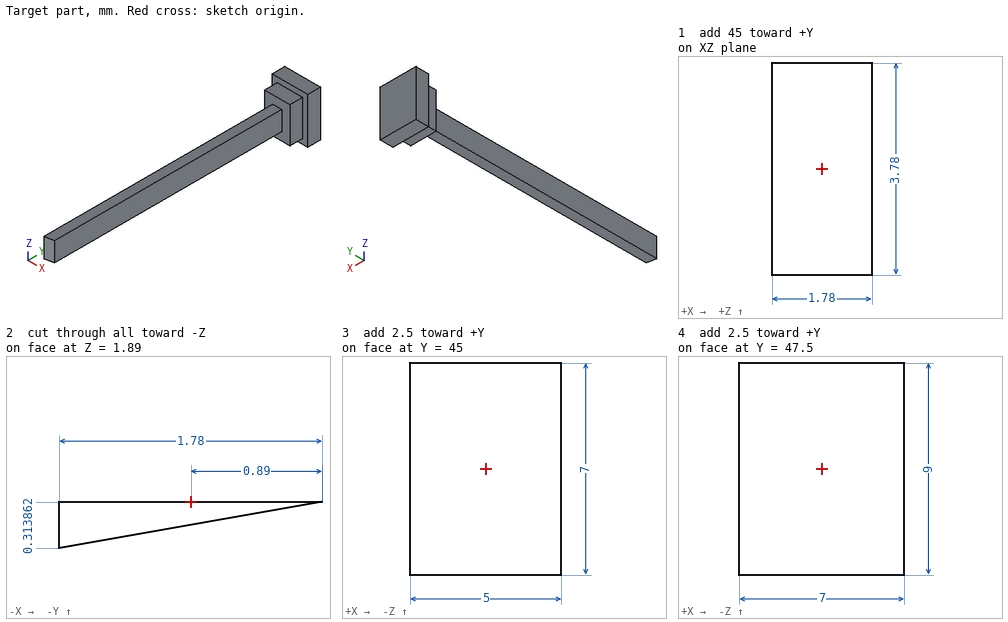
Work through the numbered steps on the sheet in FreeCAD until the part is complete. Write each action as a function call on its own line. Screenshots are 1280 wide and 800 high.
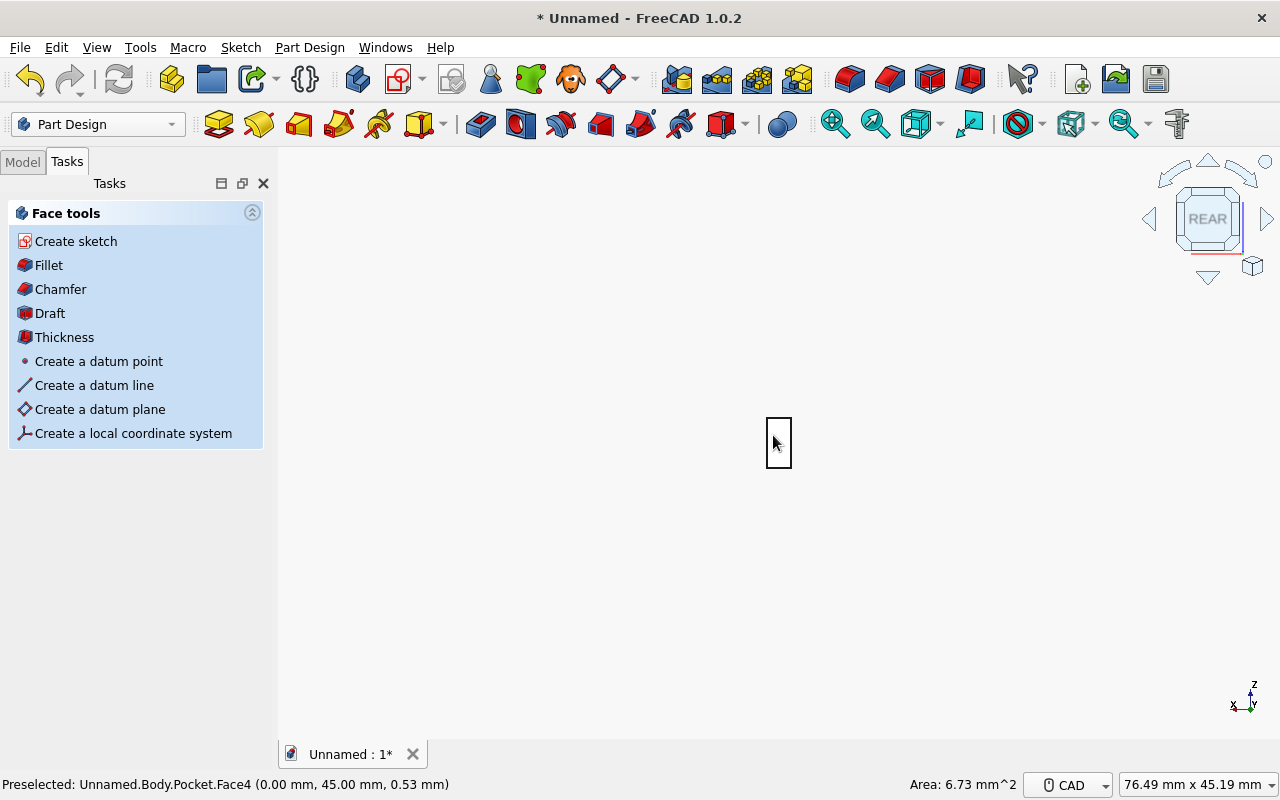
click(398, 80)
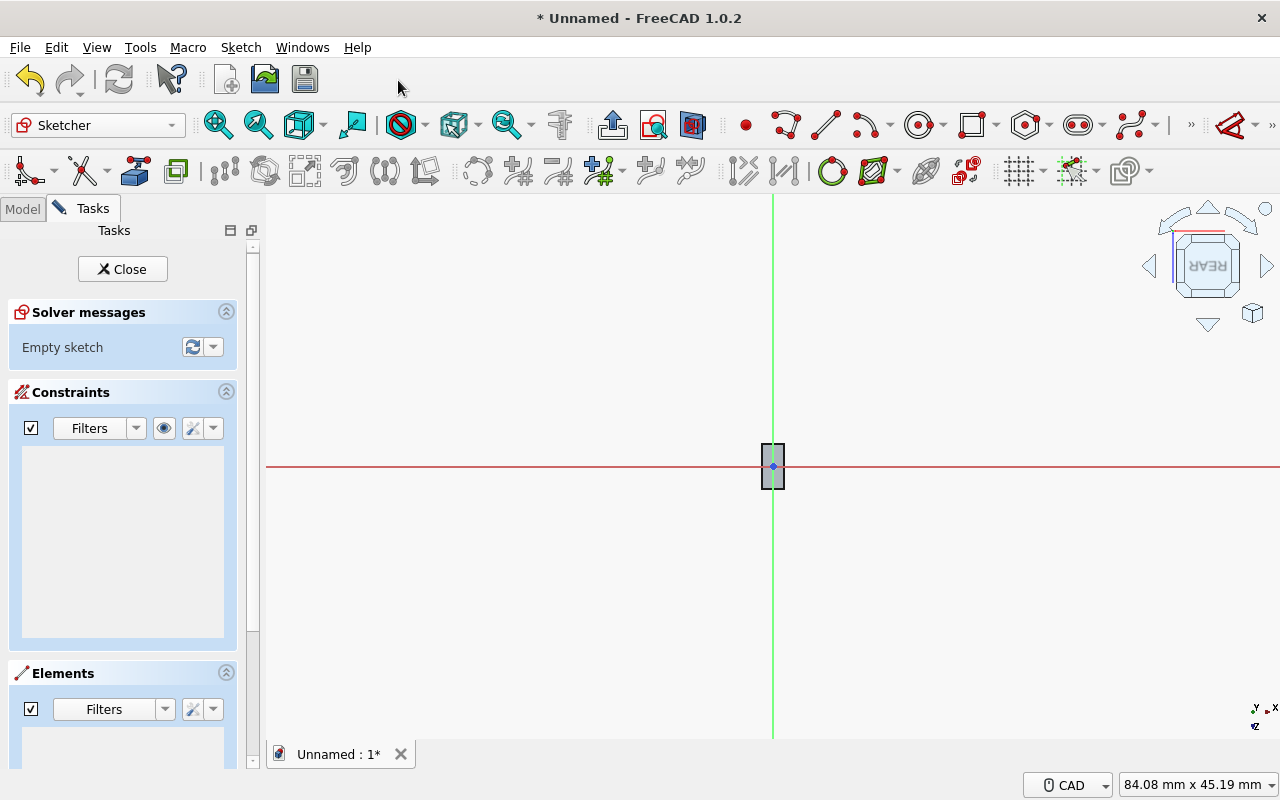
scroll(795, 466, up, 7)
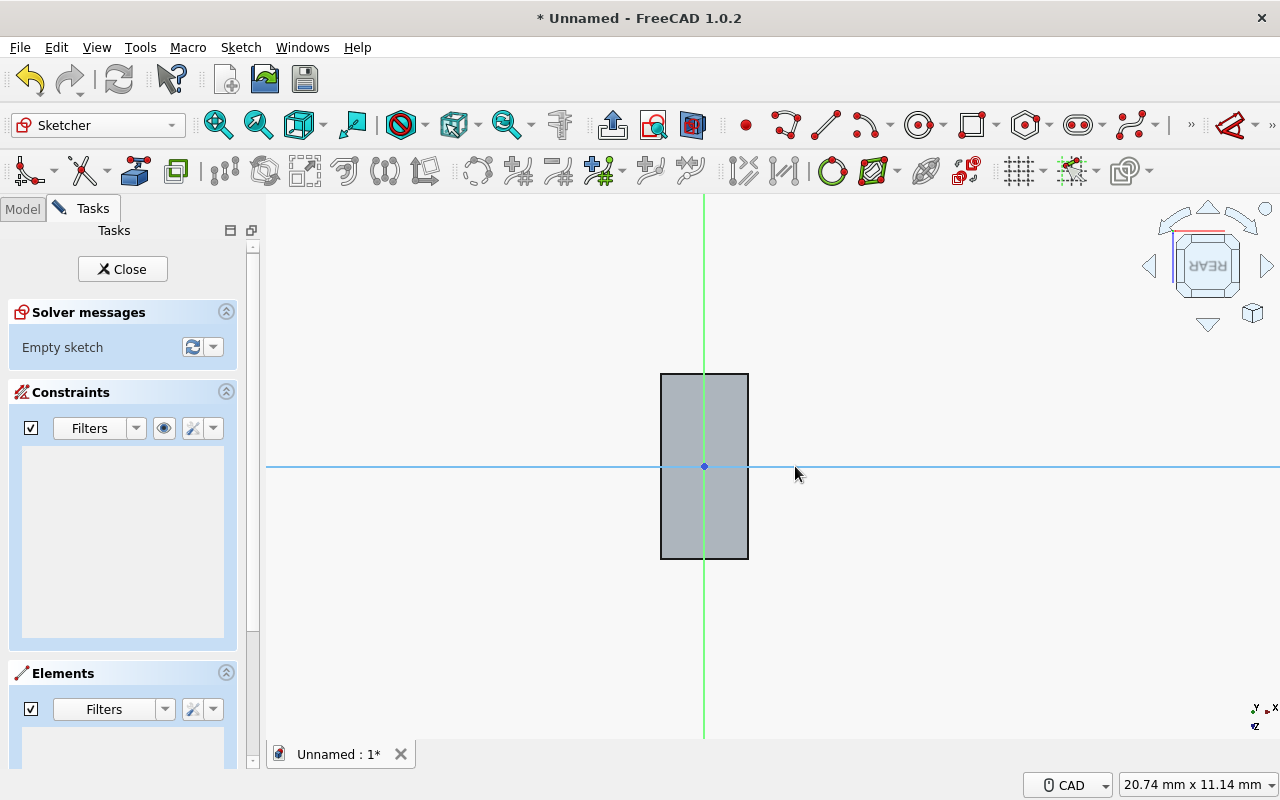
key(g)
key(v)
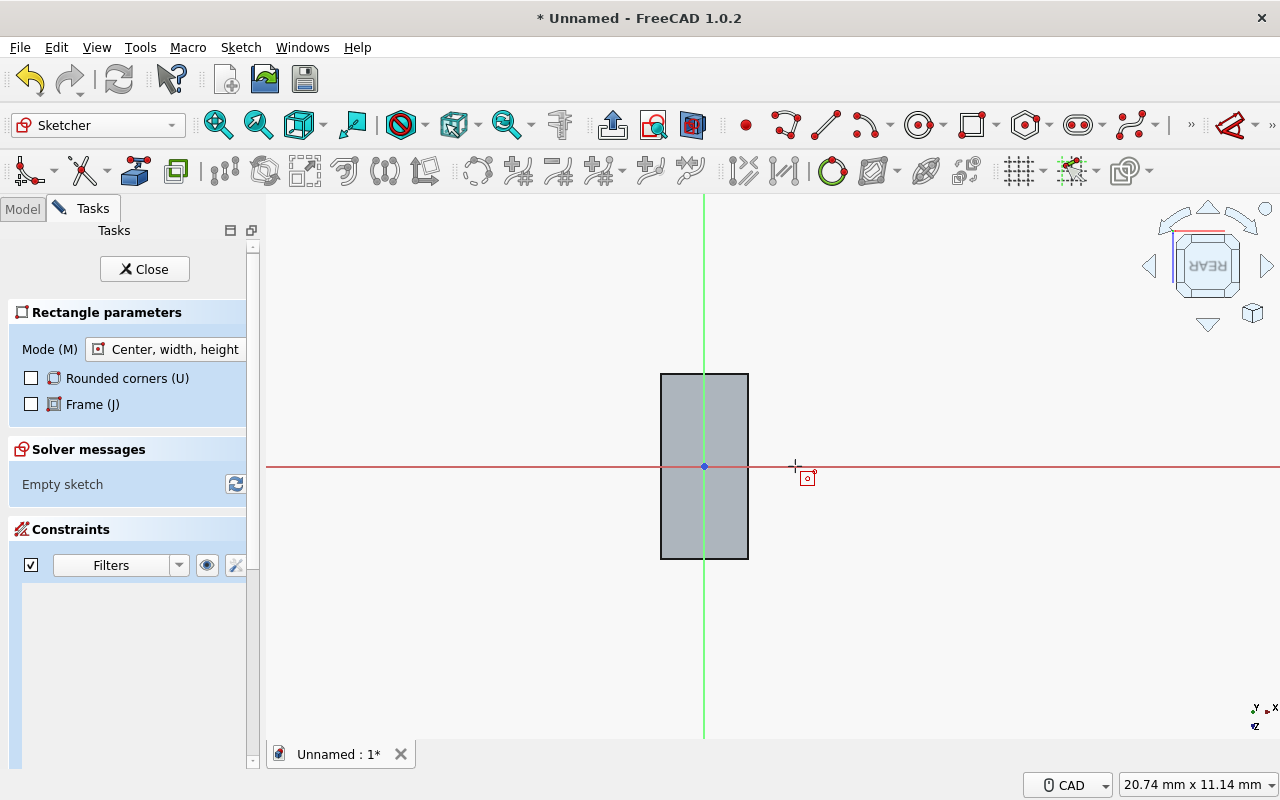
click(704, 466)
click(826, 295)
key(Escape)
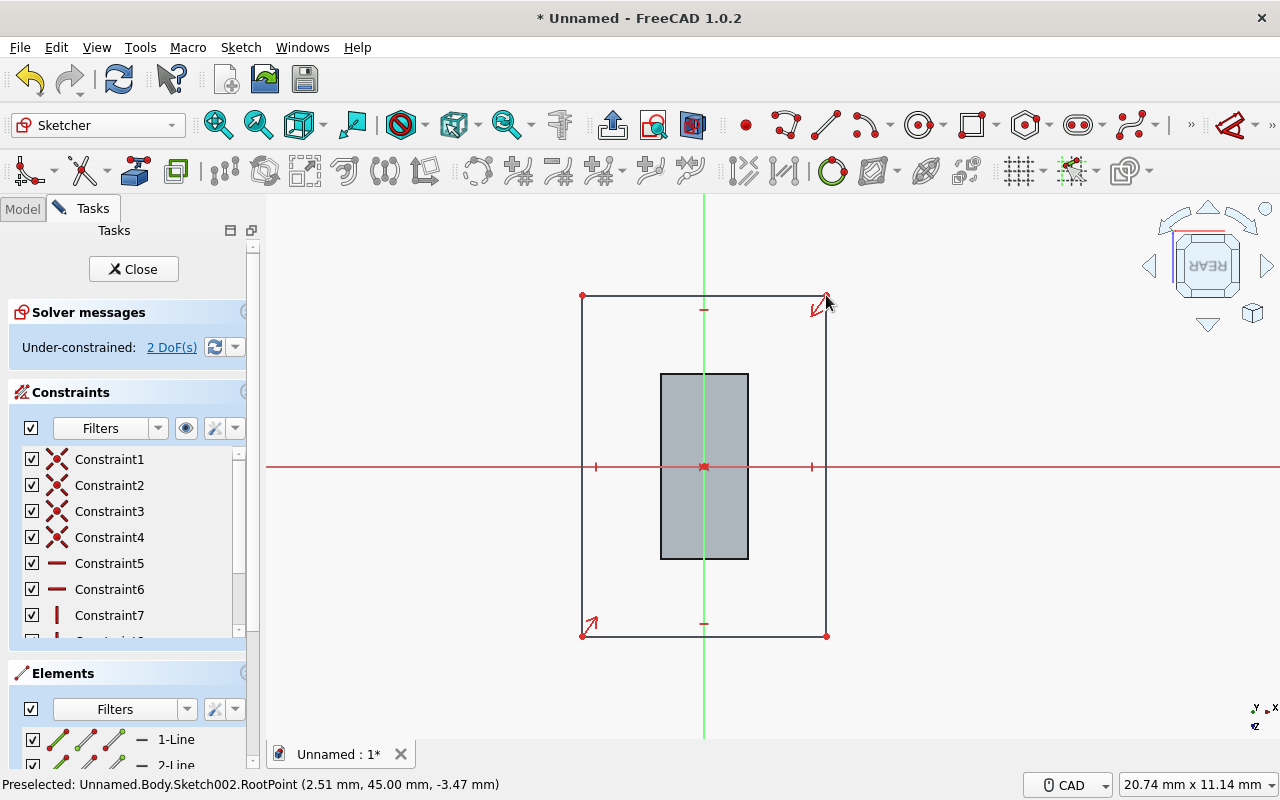
click(1230, 126)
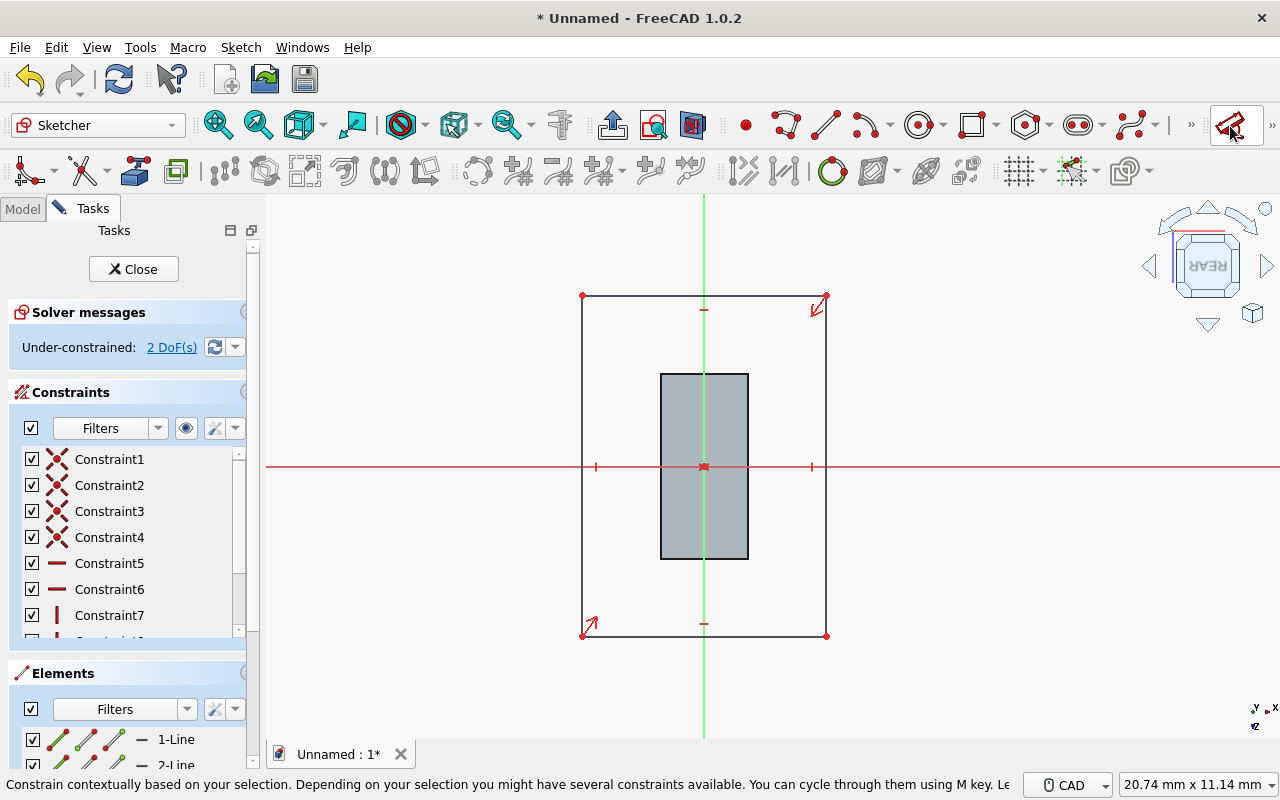
click(655, 637)
click(648, 671)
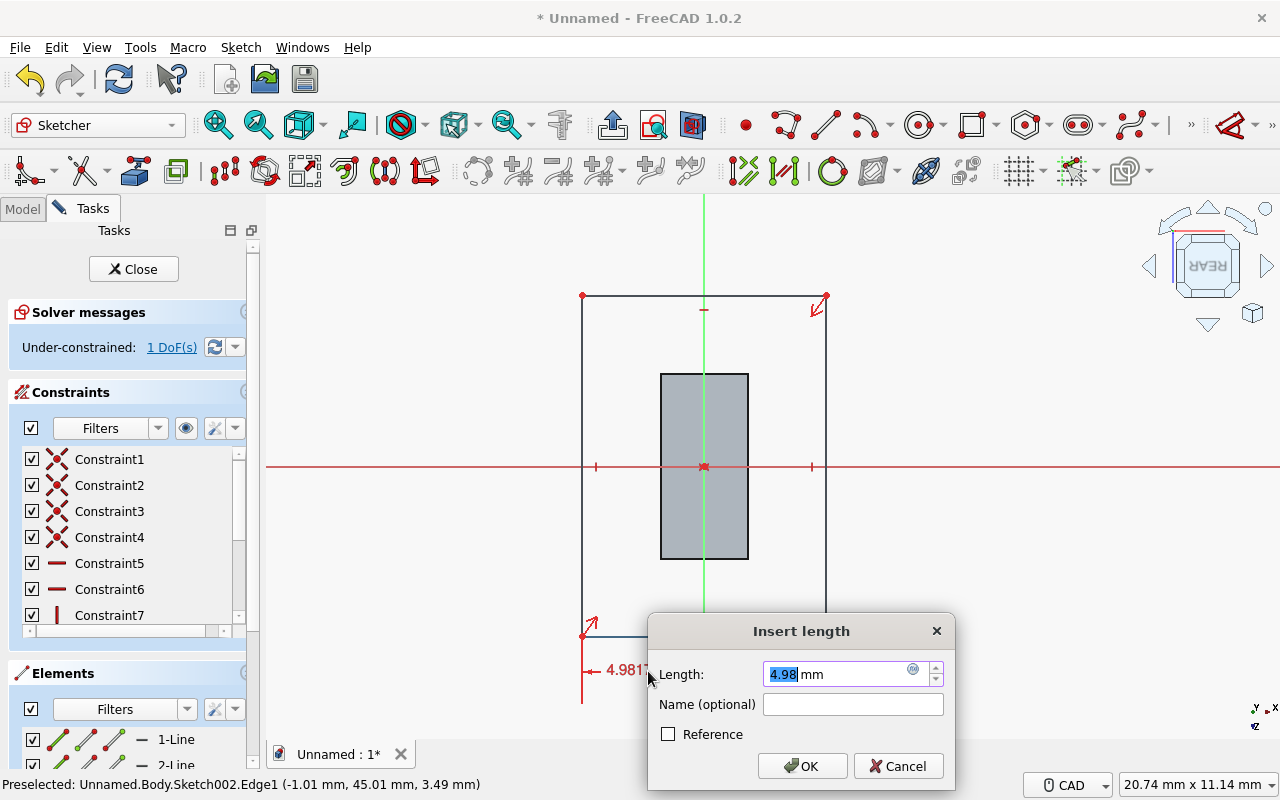
text(5)
key(Return)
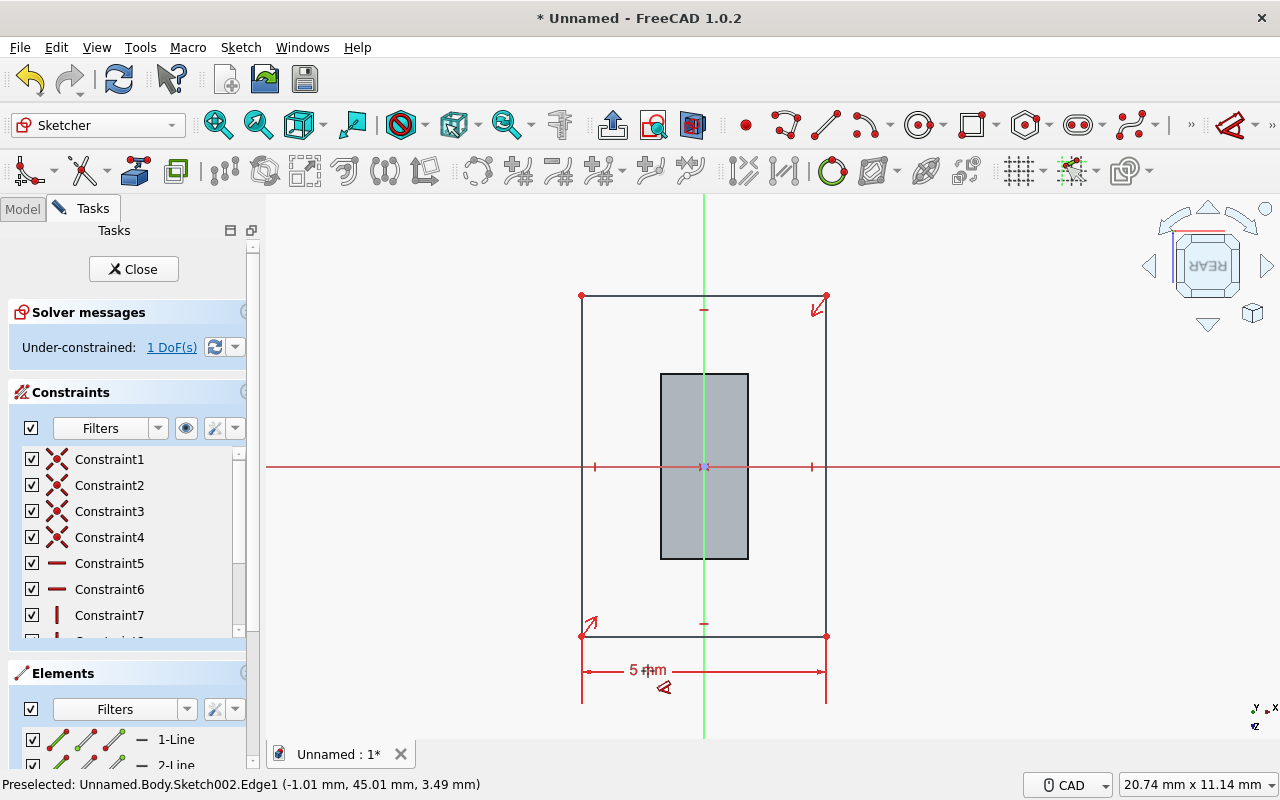
click(826, 535)
click(860, 388)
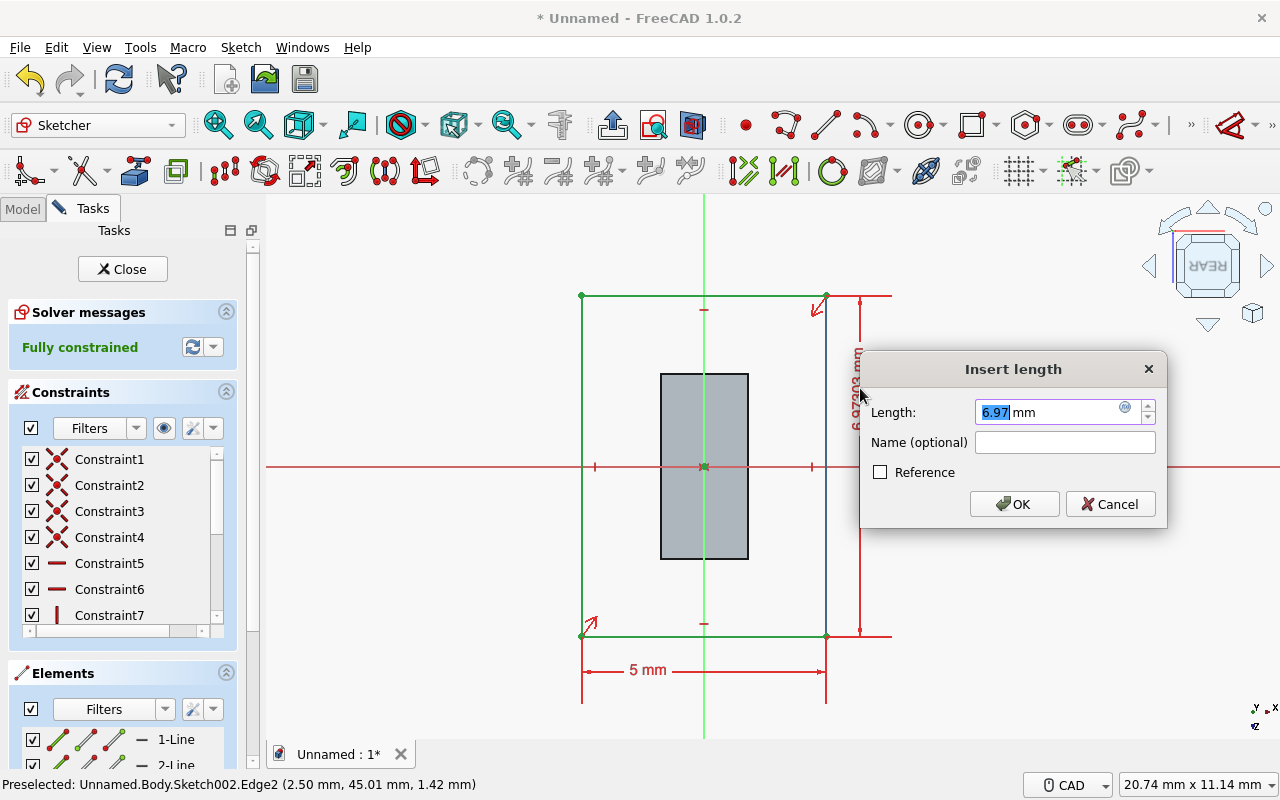
text(7)
key(Return)
key(Escape)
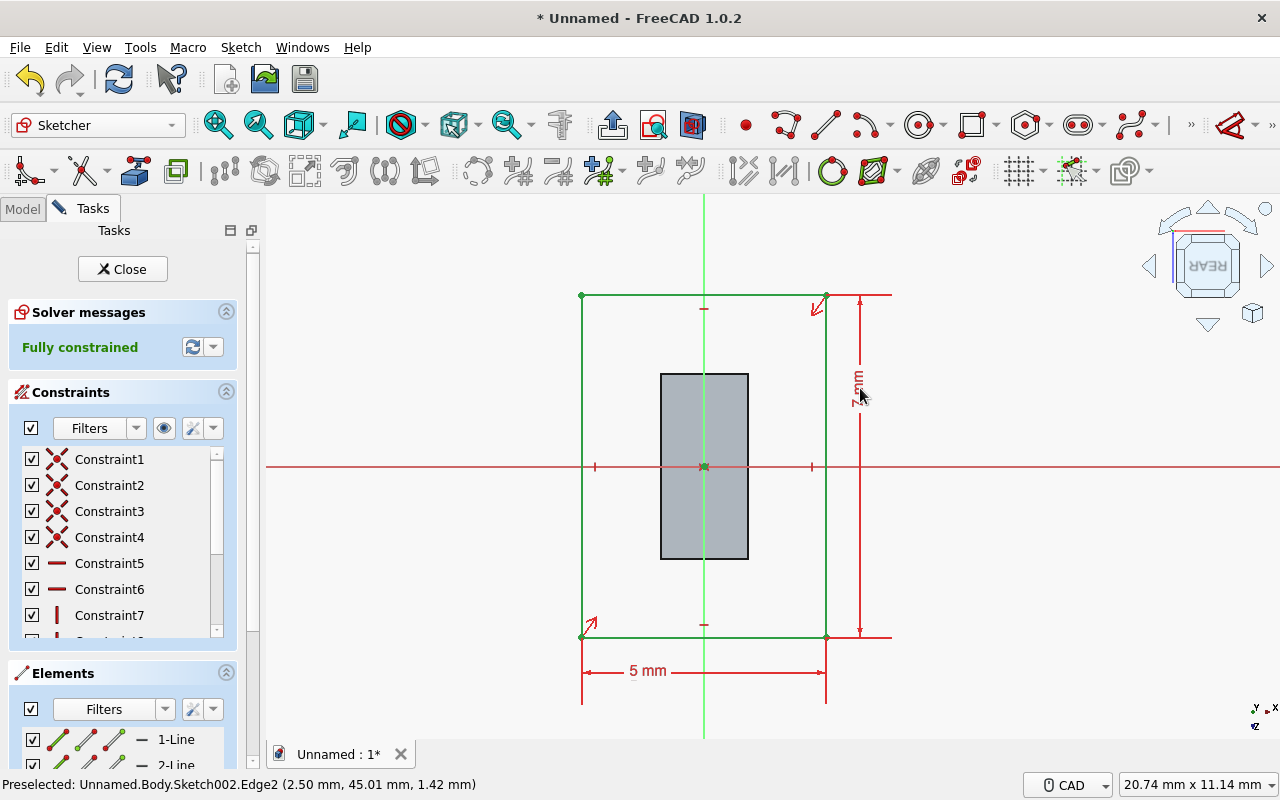
click(123, 269)